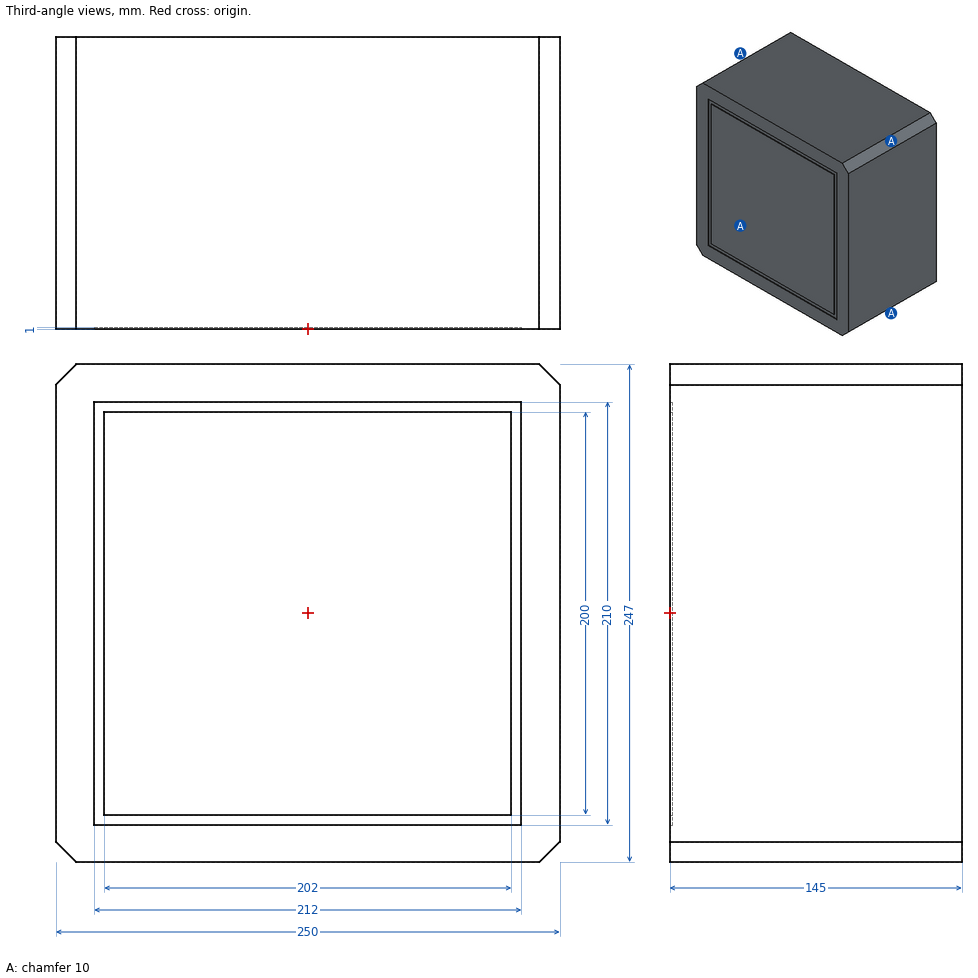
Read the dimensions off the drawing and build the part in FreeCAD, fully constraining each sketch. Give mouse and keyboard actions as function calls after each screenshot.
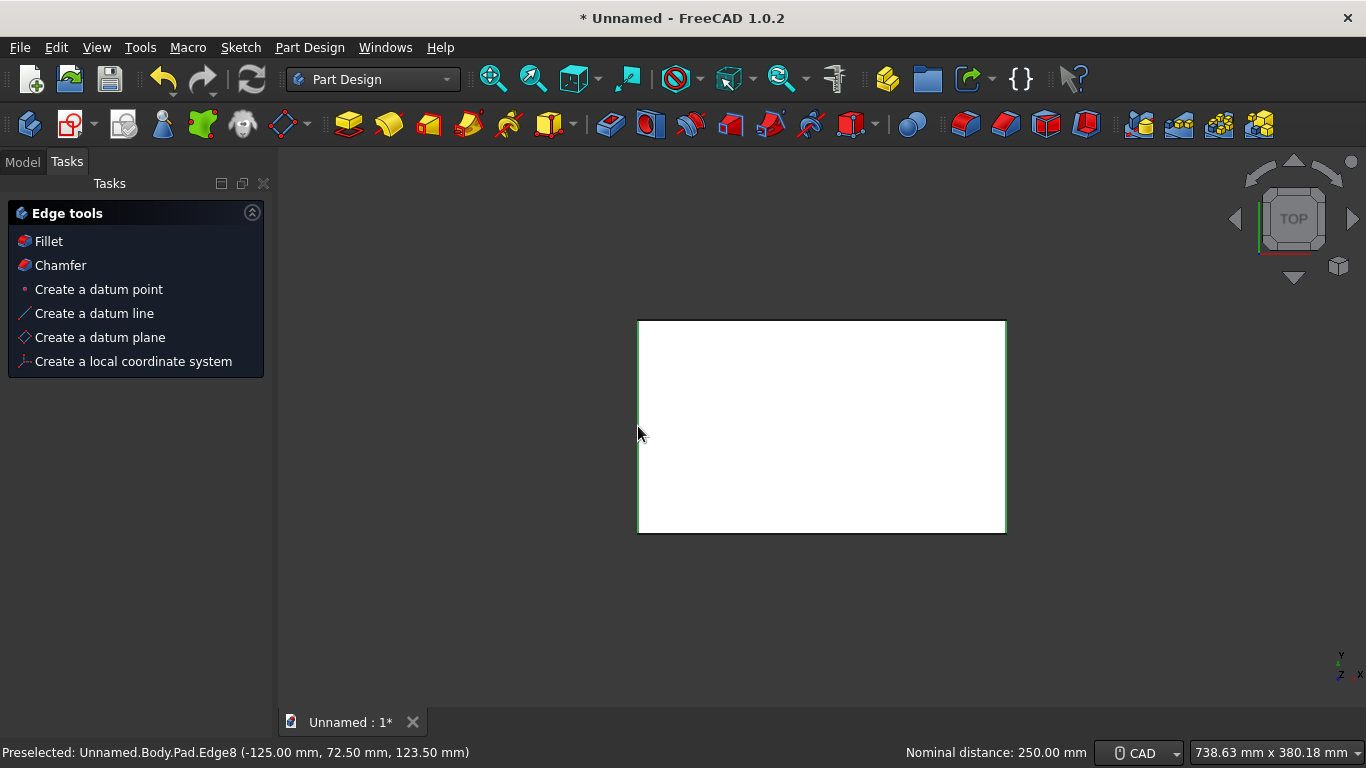
key(1)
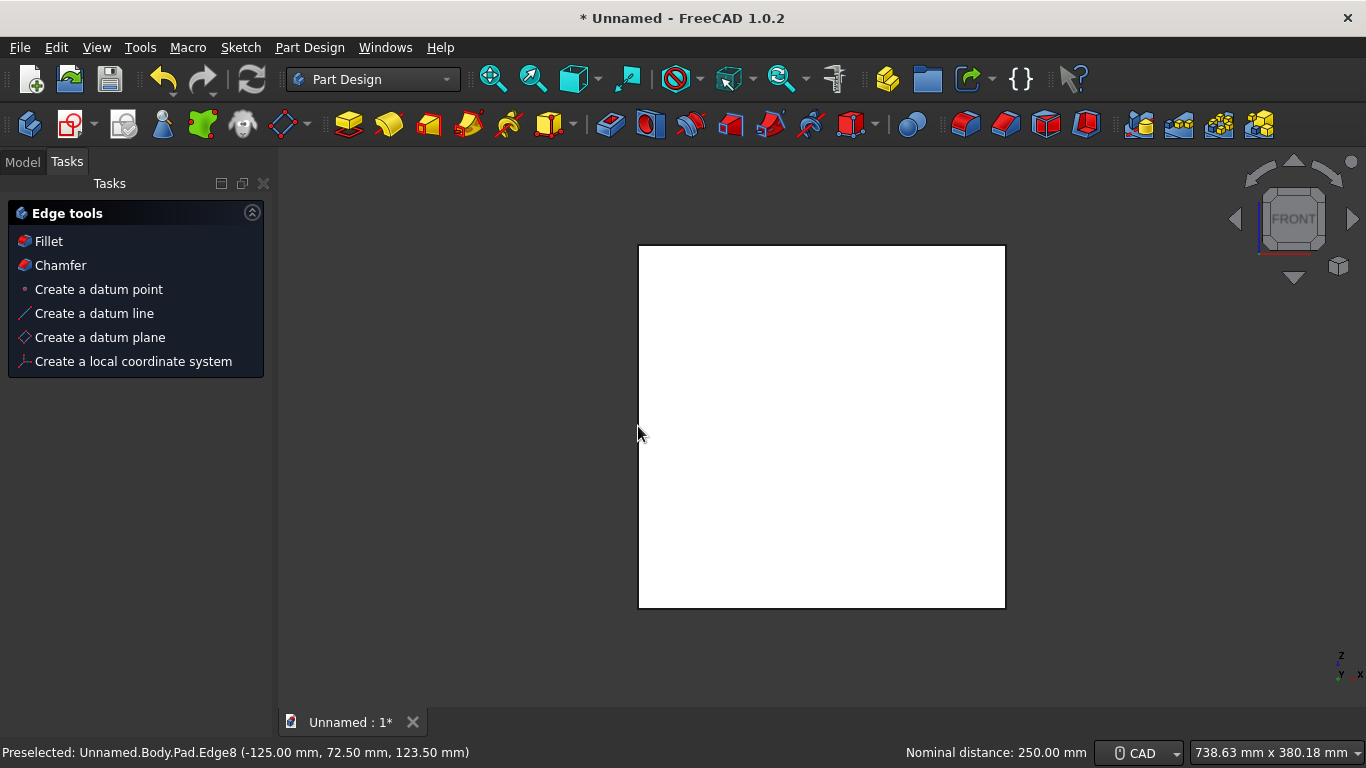
key(3)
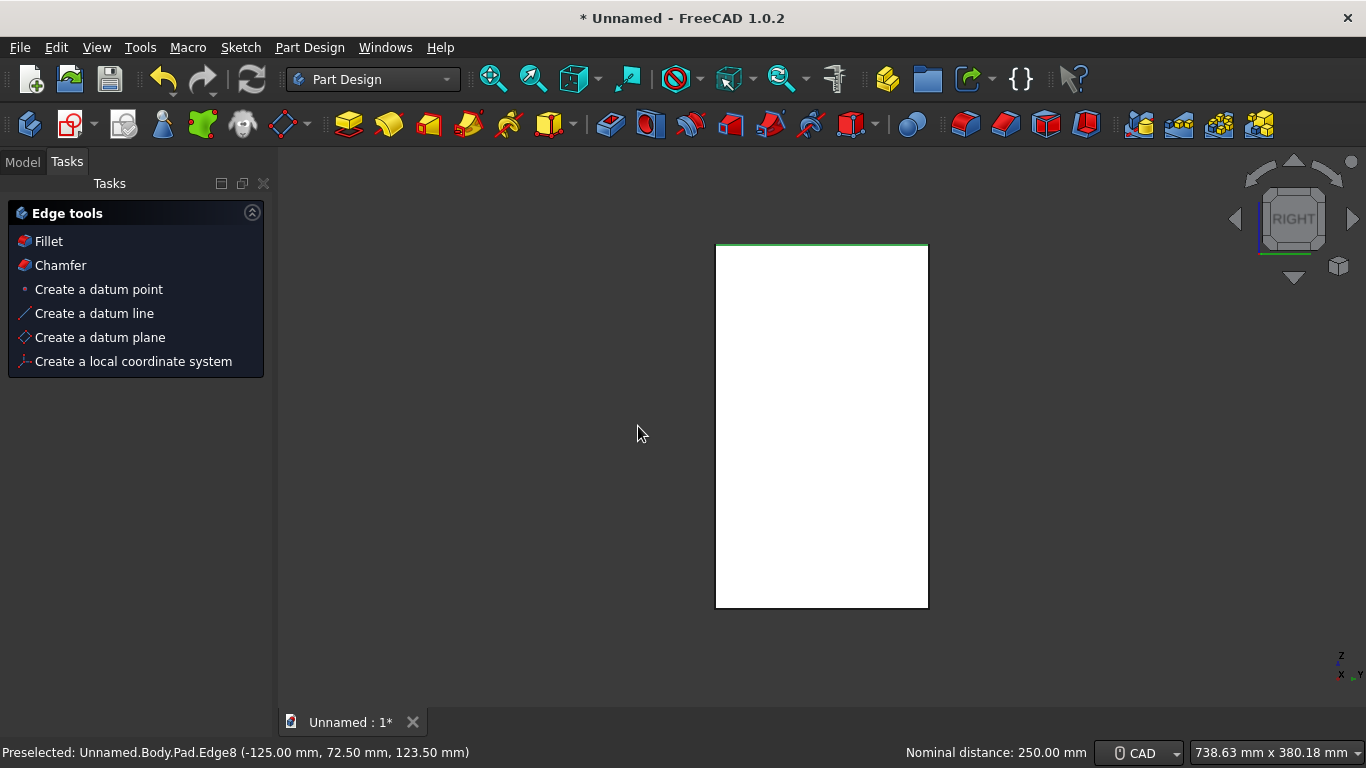
click(822, 608, ctrl)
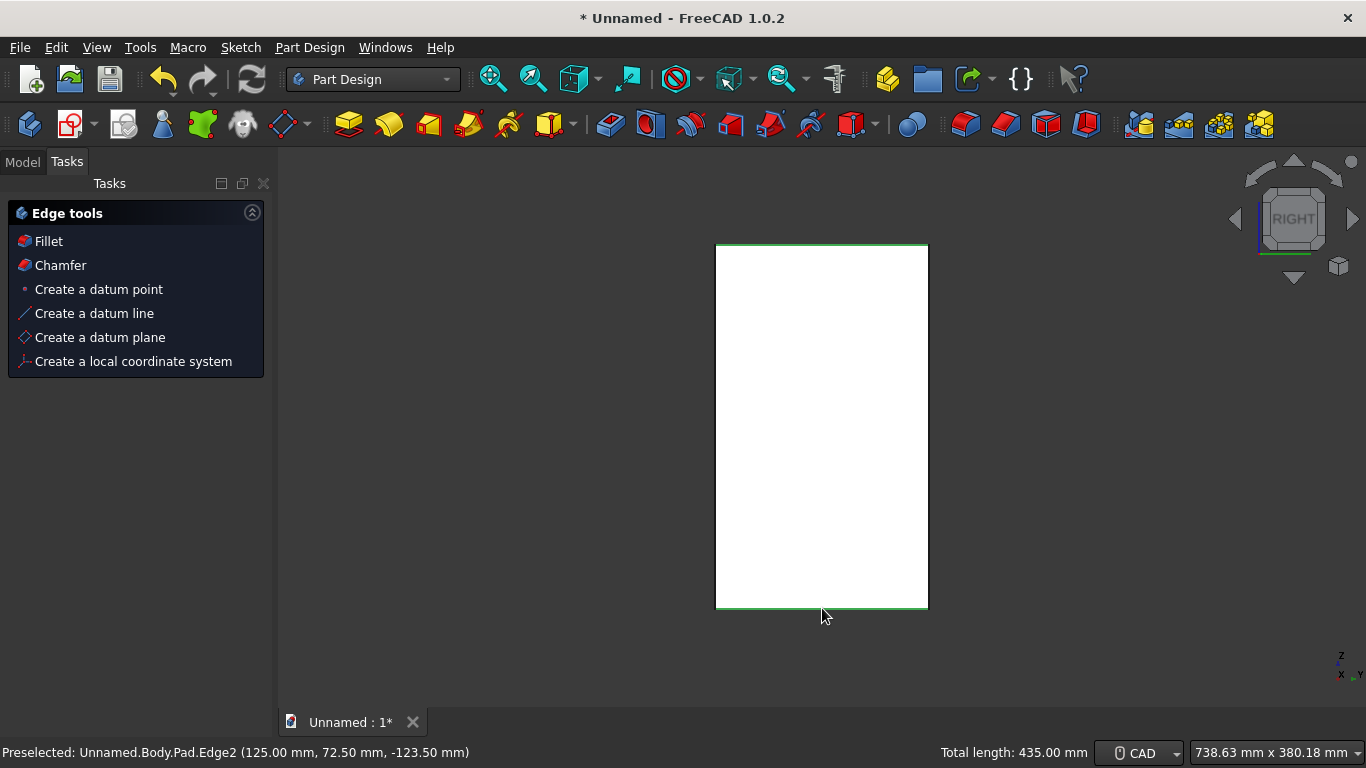
key(5)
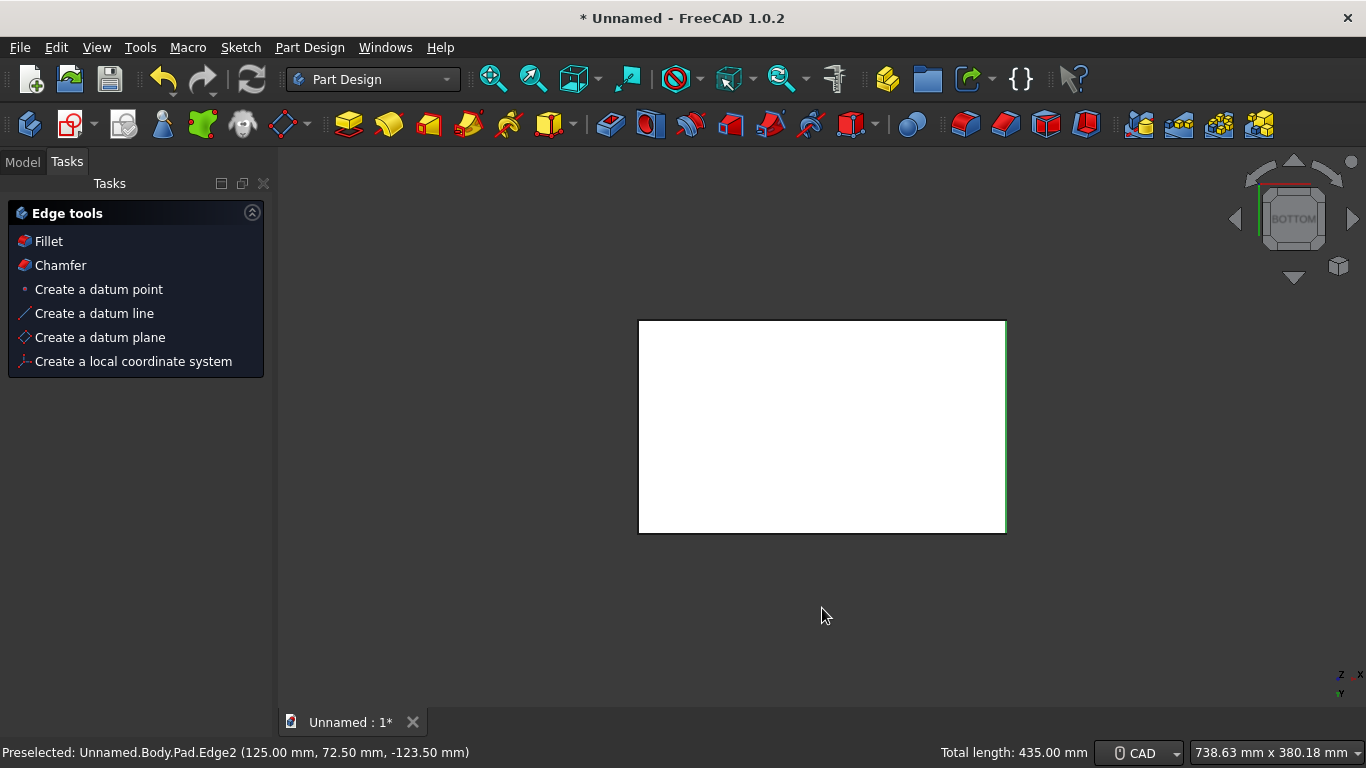
key(v)
key(f)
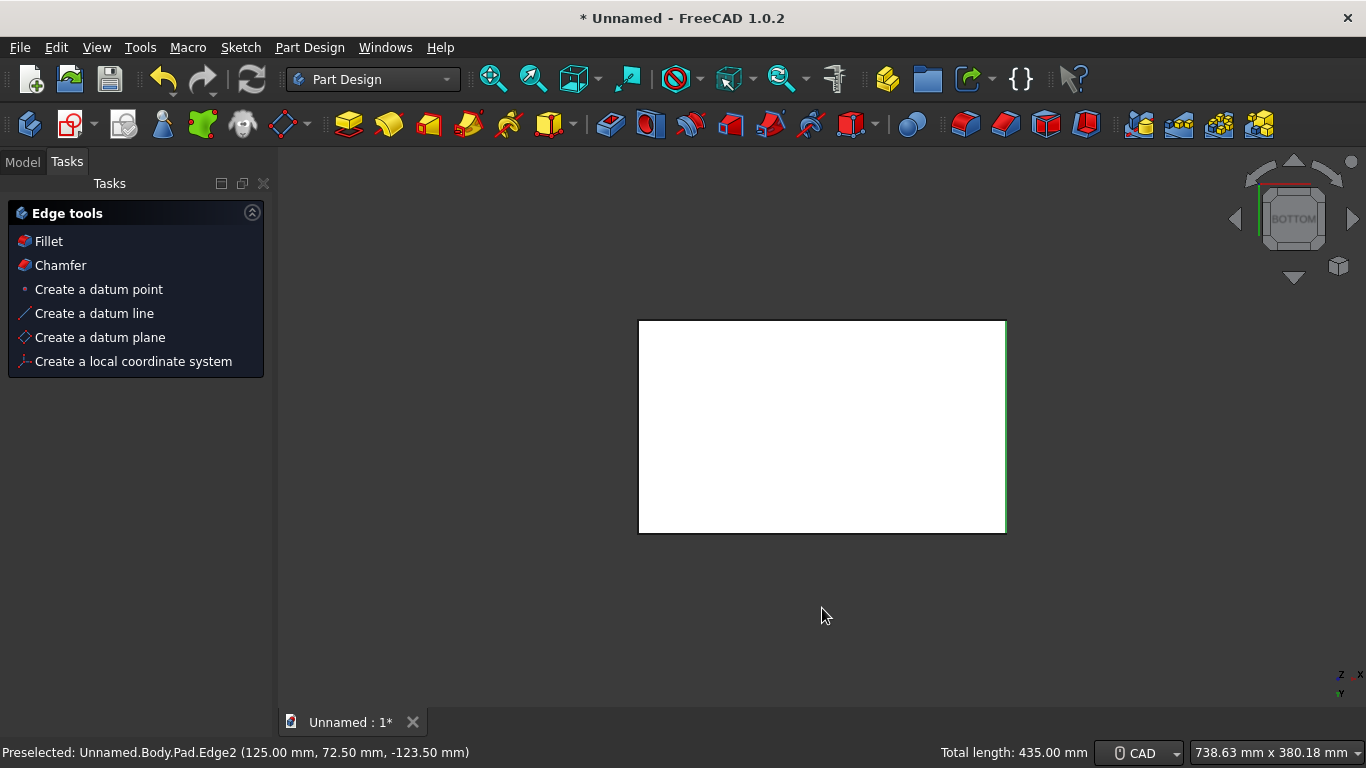
click(638, 426, ctrl)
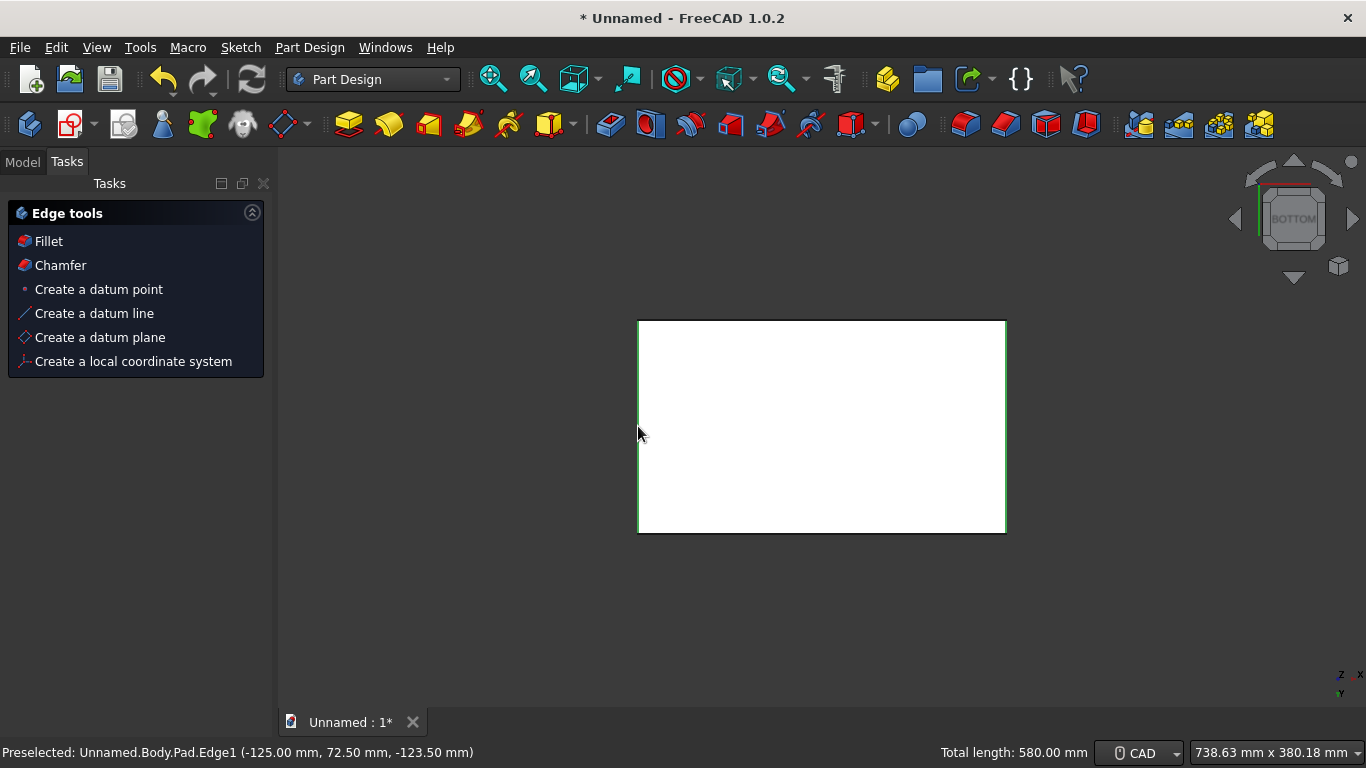
click(1006, 124)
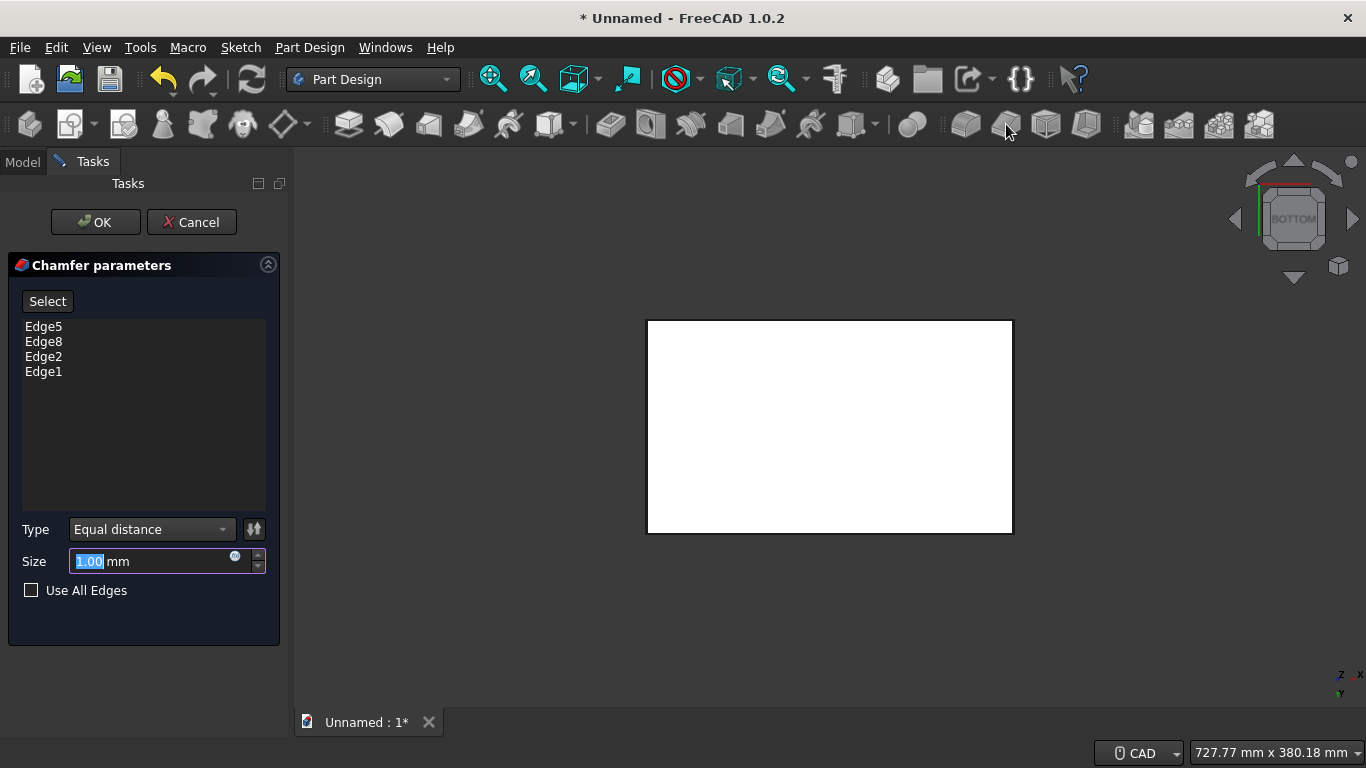
text(10)
key(Tab)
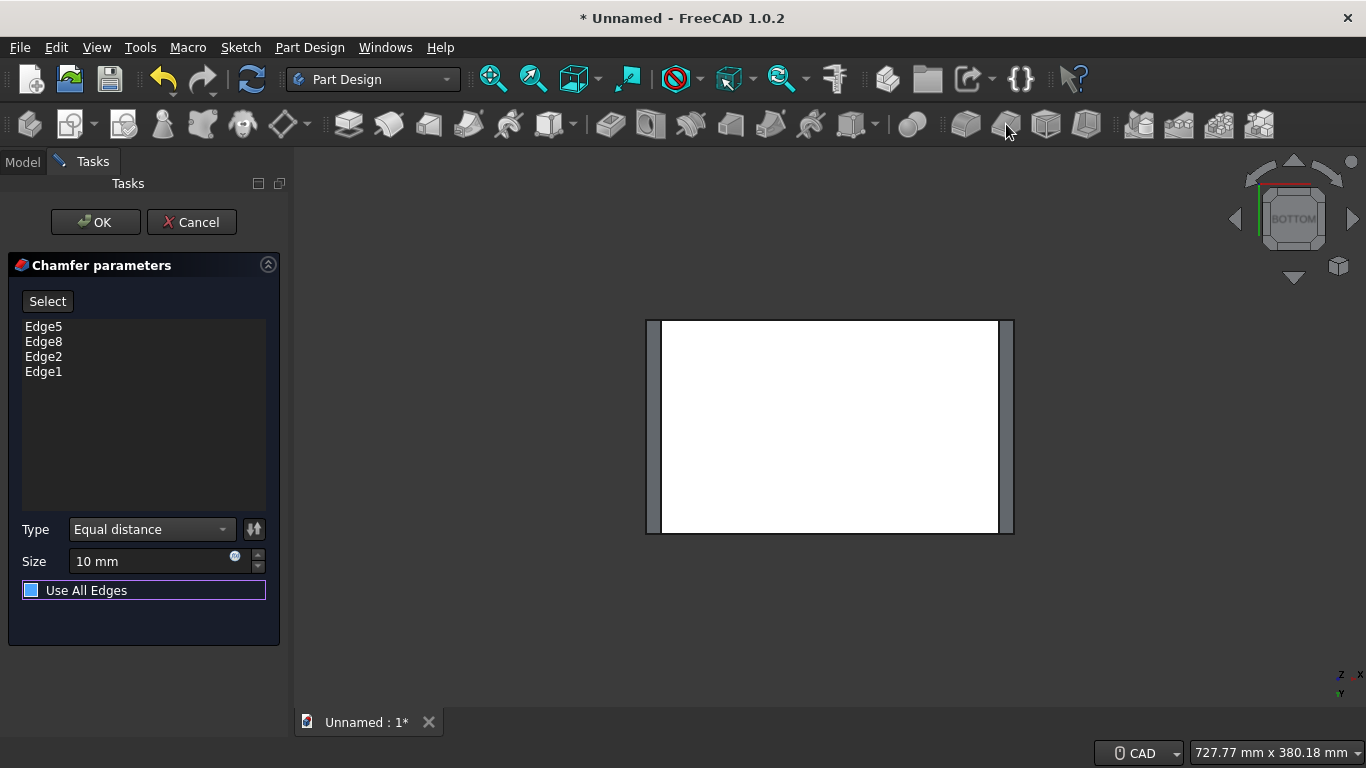
click(96, 222)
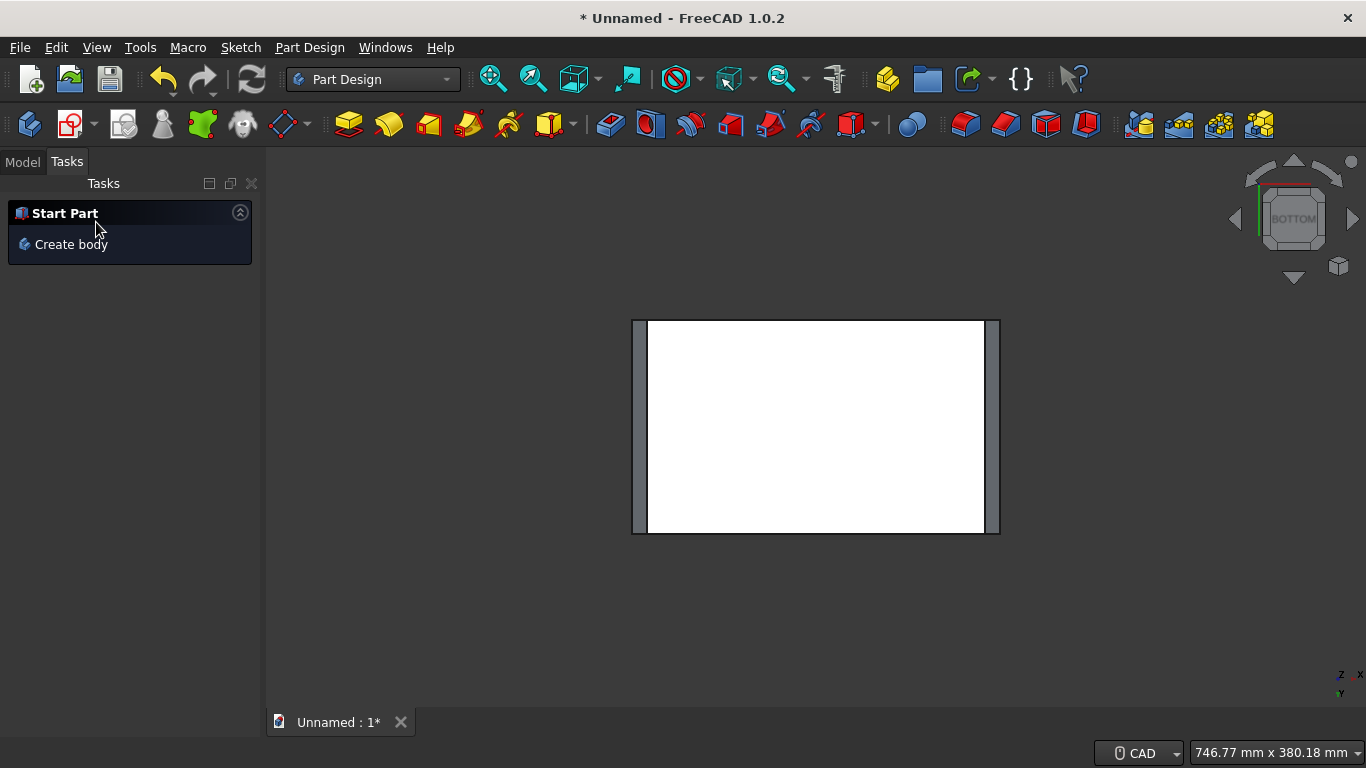
key(v)
key(f)